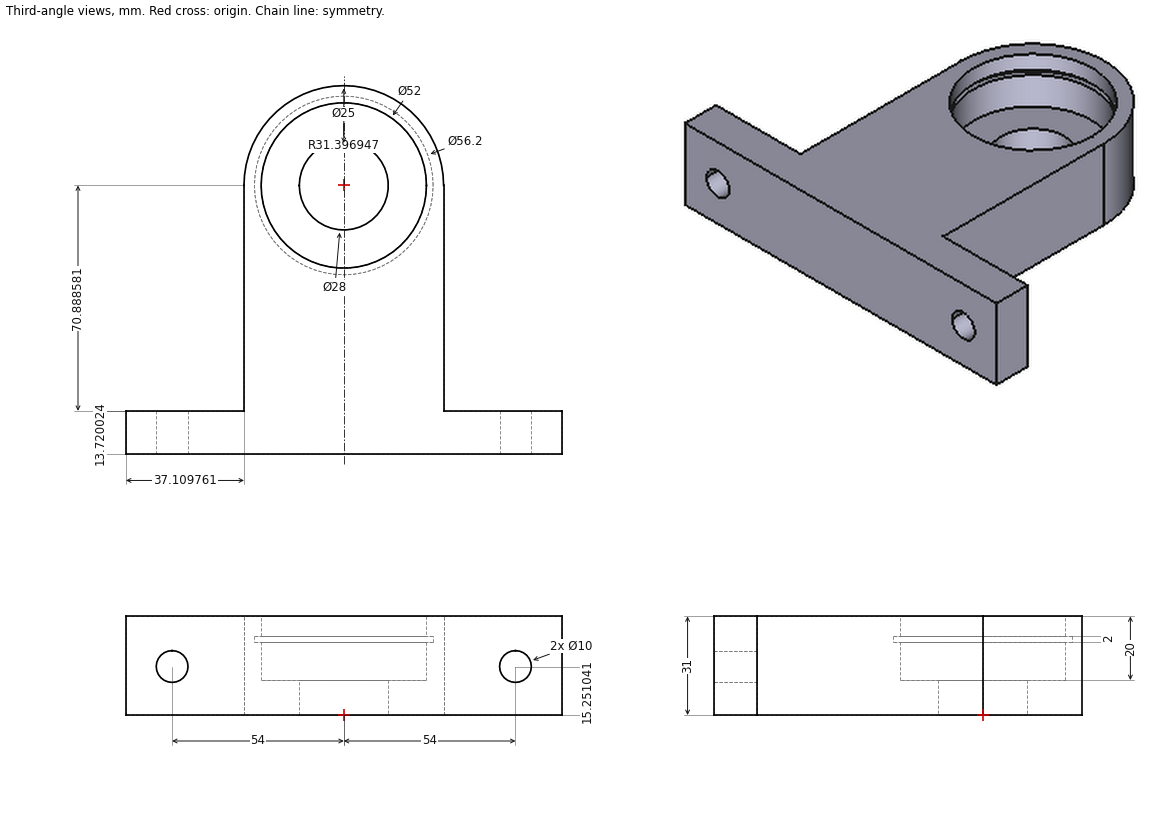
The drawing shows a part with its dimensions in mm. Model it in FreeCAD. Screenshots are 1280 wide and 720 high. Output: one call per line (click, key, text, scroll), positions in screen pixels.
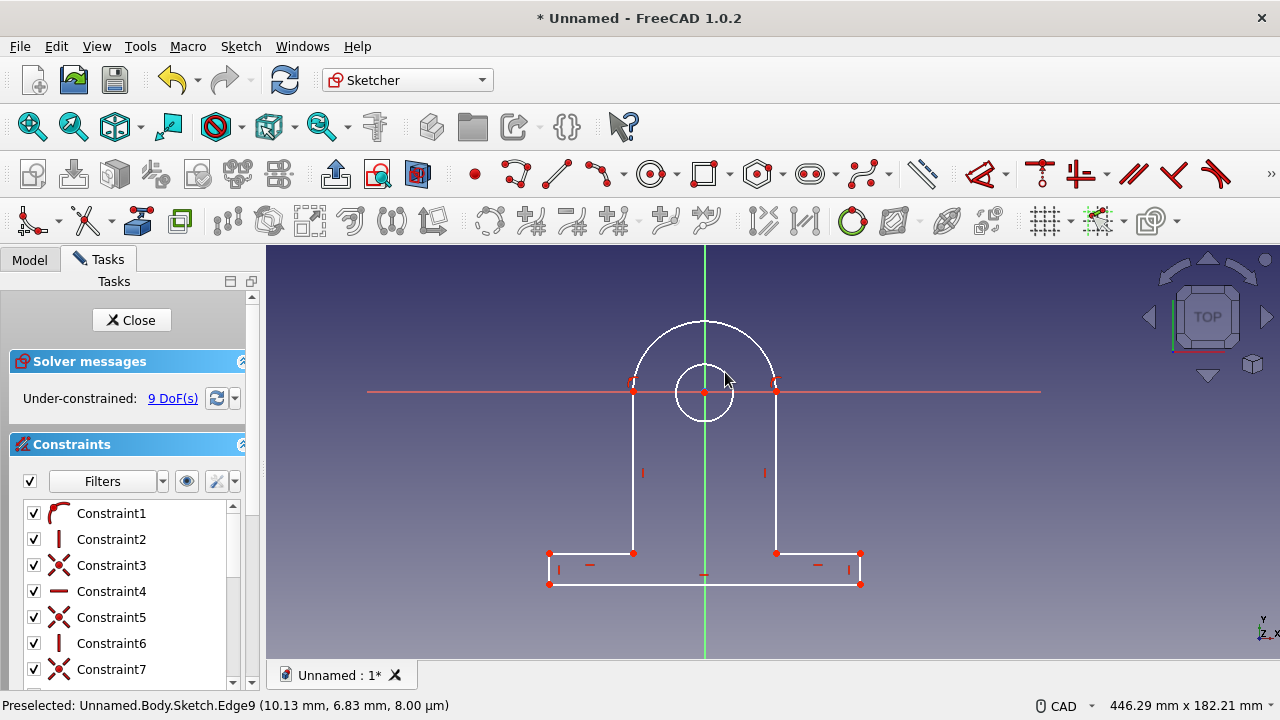
scroll(705, 392, up, 2)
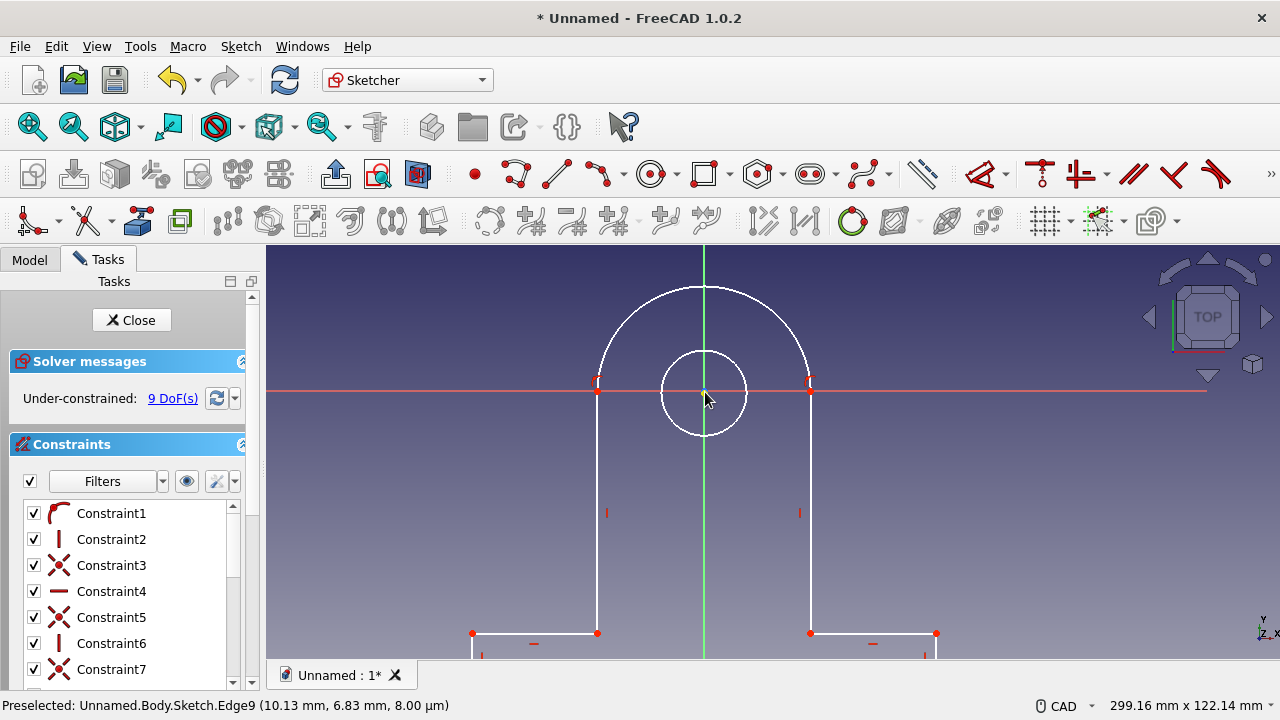
drag(694, 381, 714, 403)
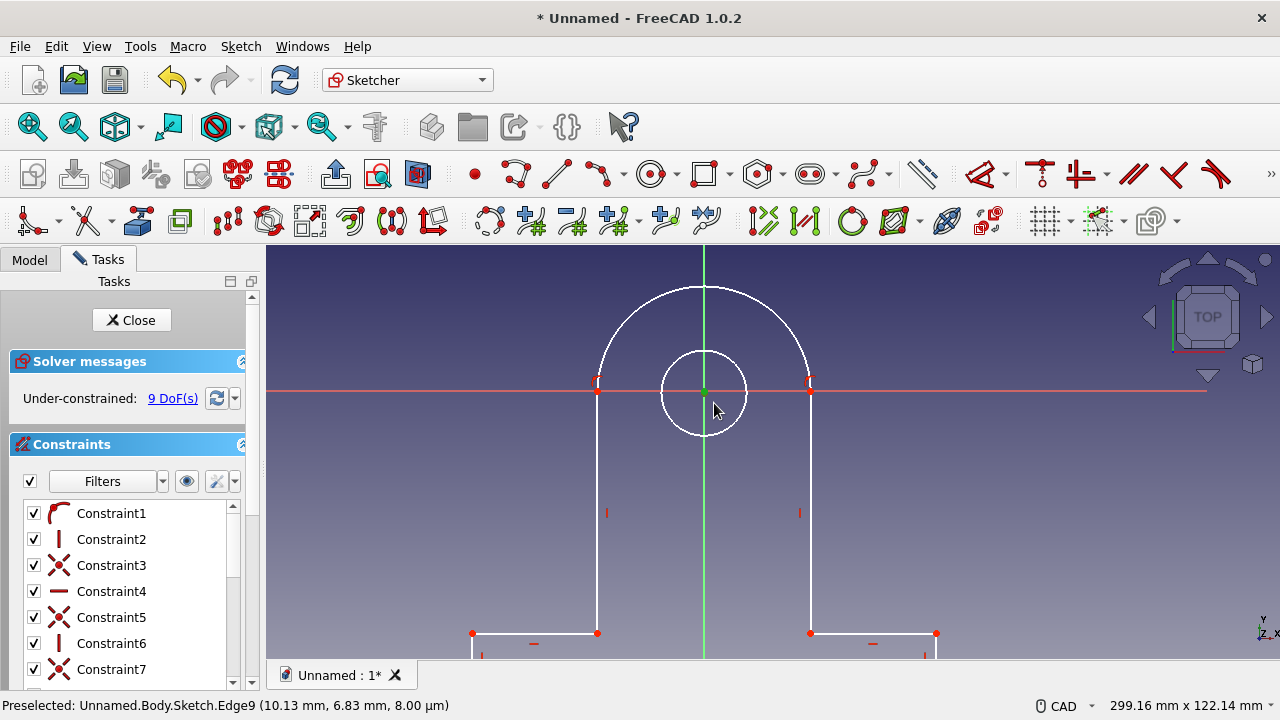
click(1040, 174)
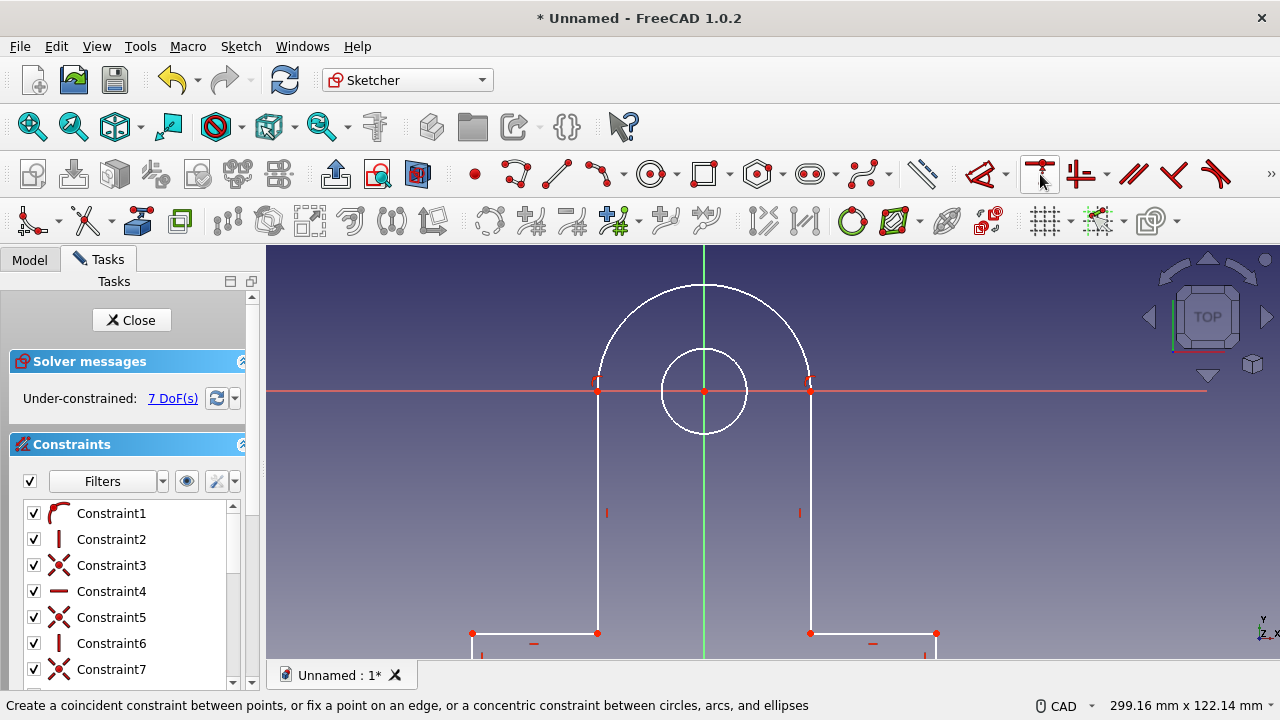
scroll(705, 392, down, 2)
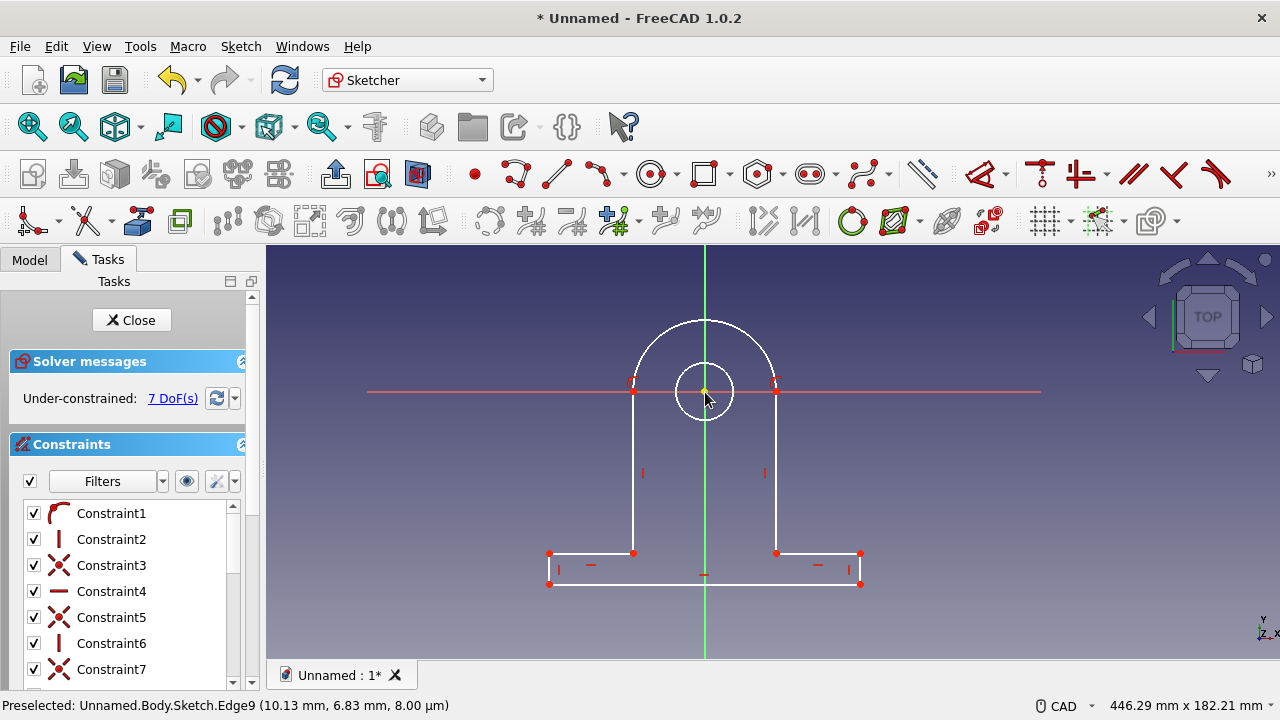
click(549, 554)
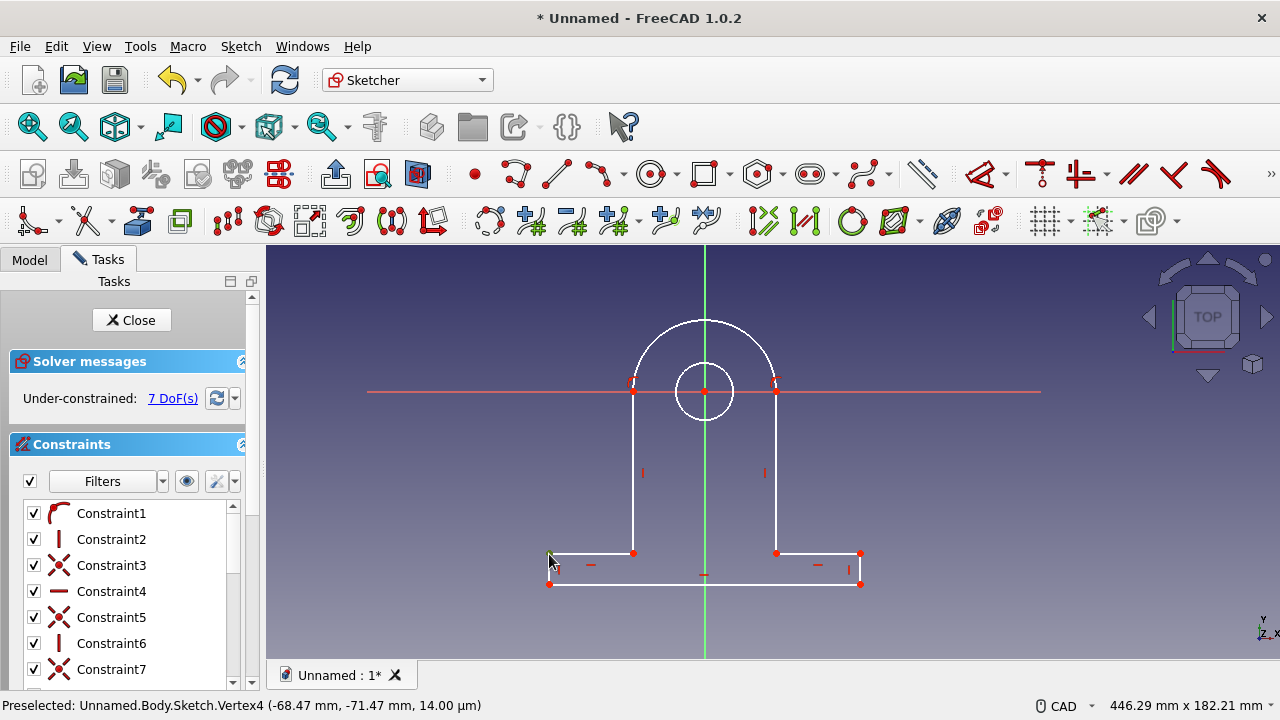
click(860, 554)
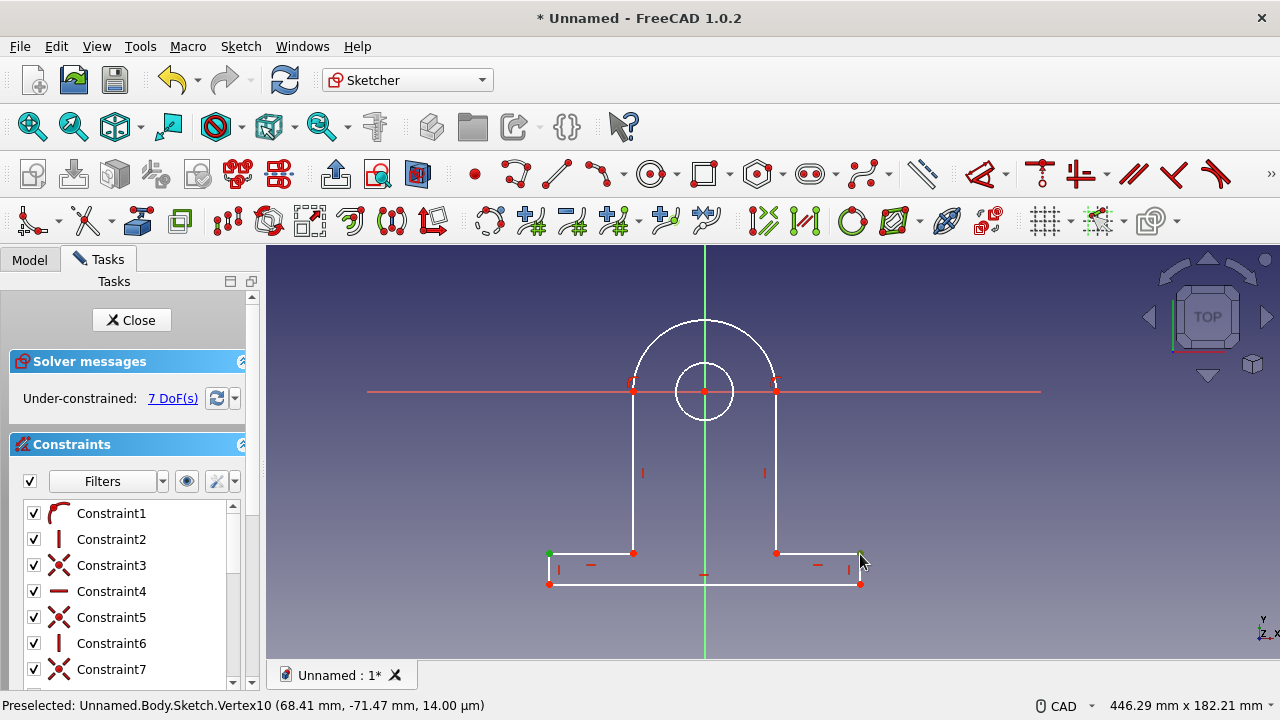
click(705, 554)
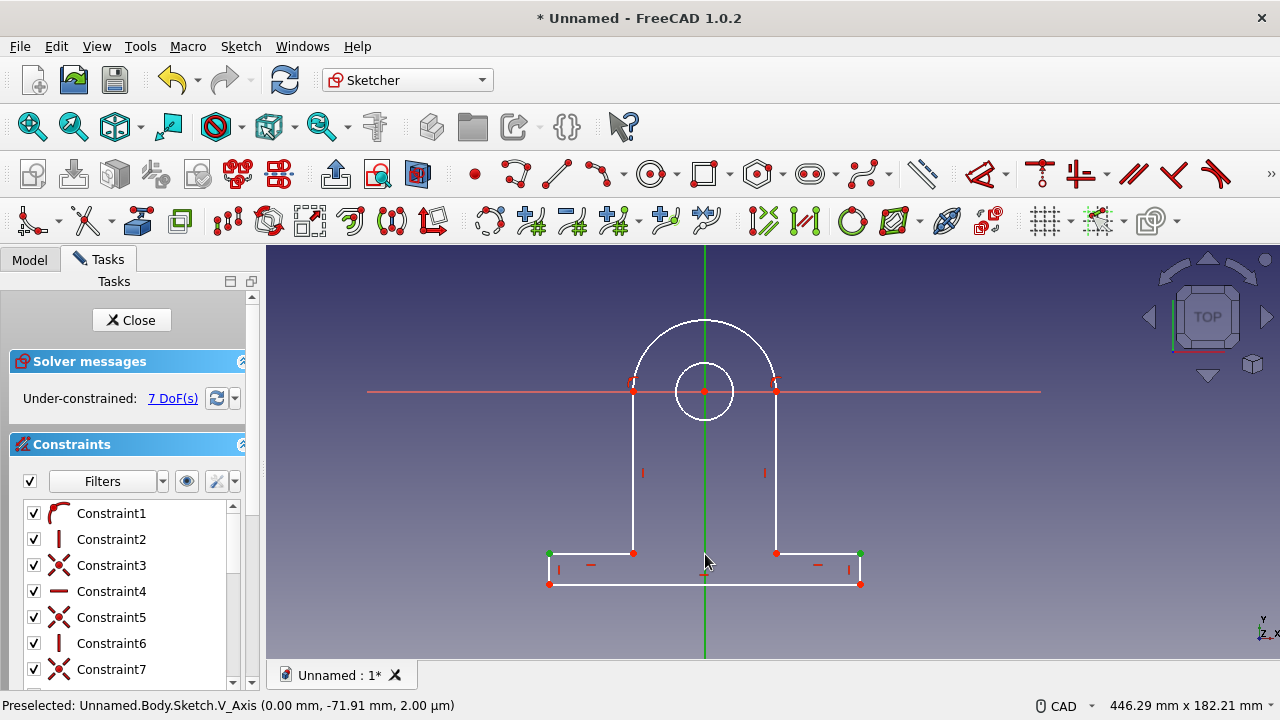
key(s)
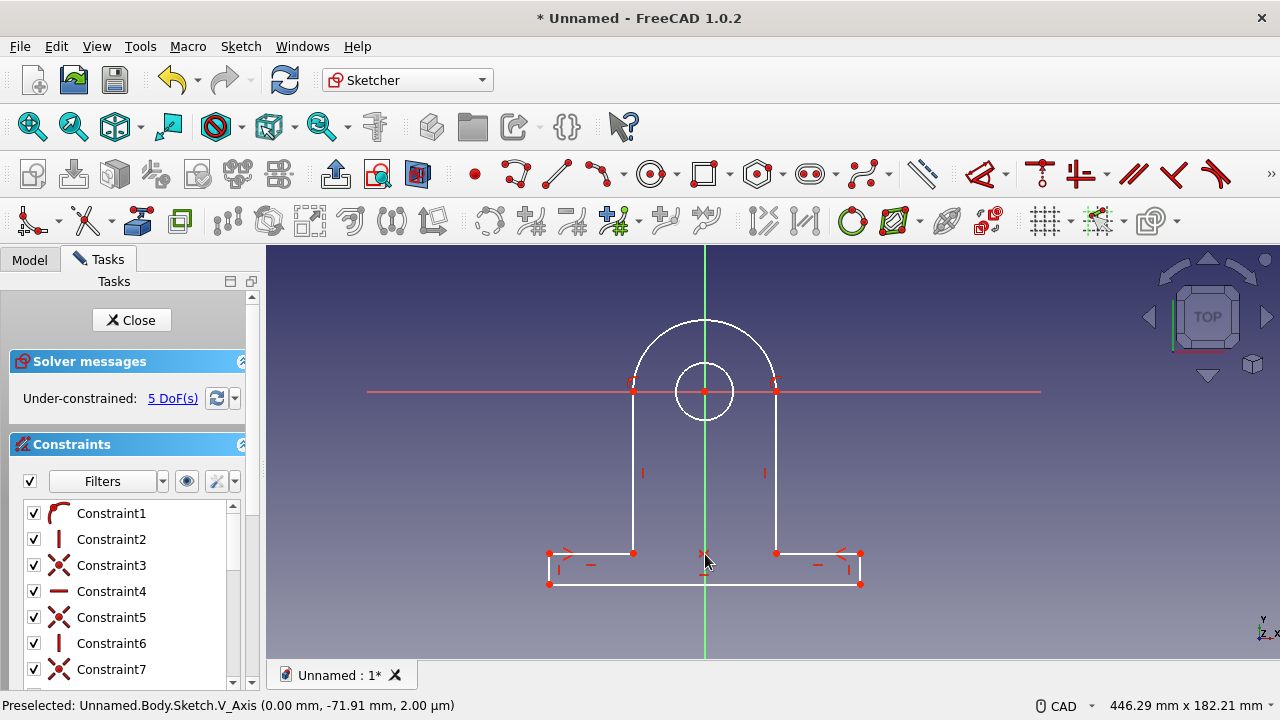
key(d)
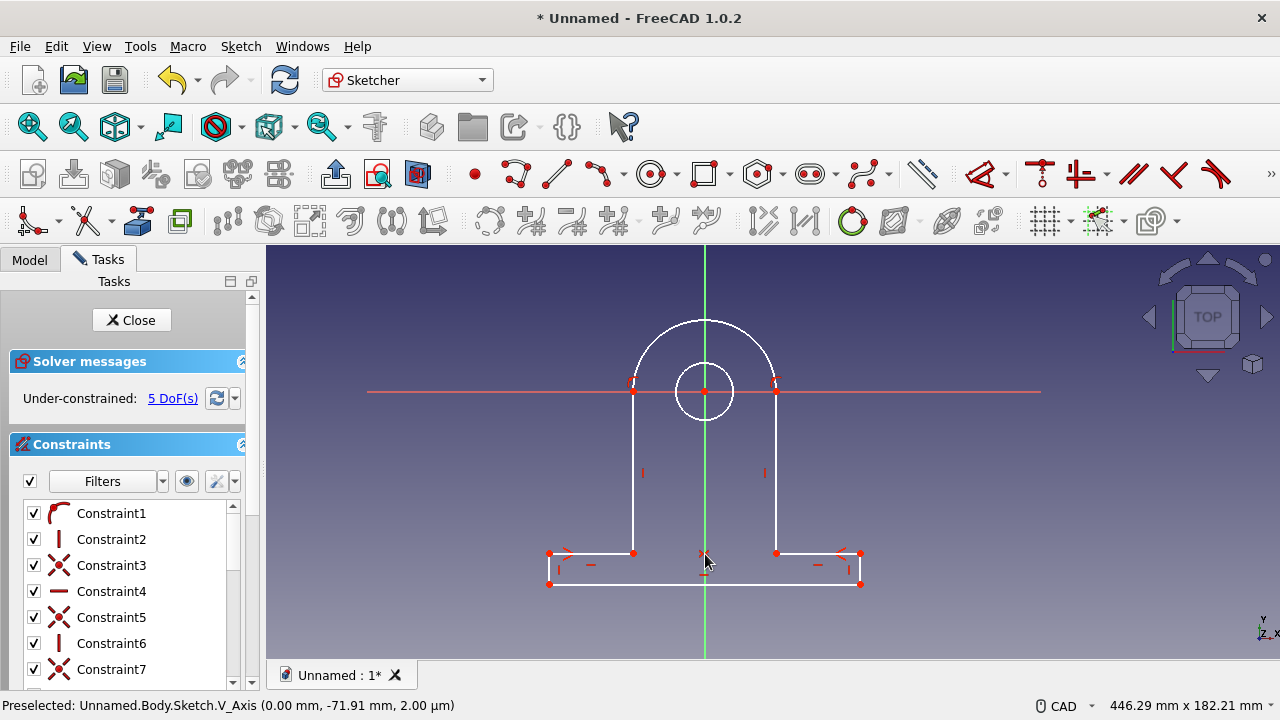
click(747, 334)
click(766, 308)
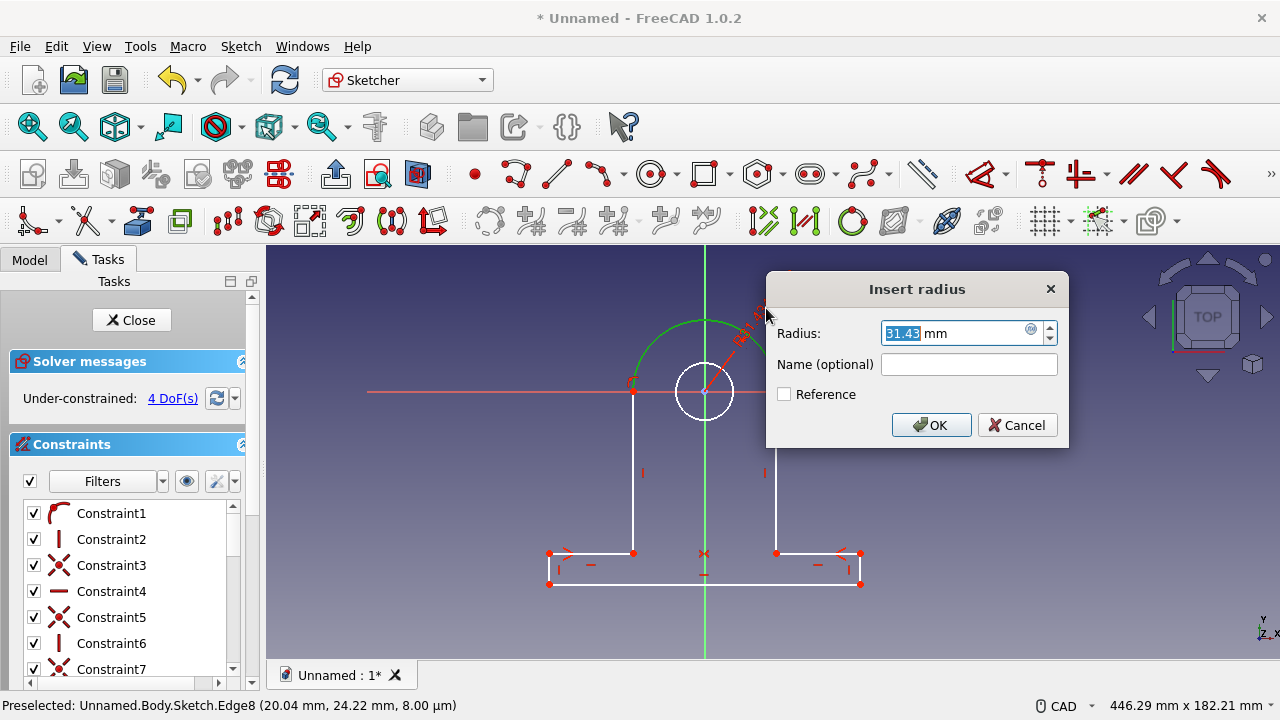
text(31.396947)
key(Return)